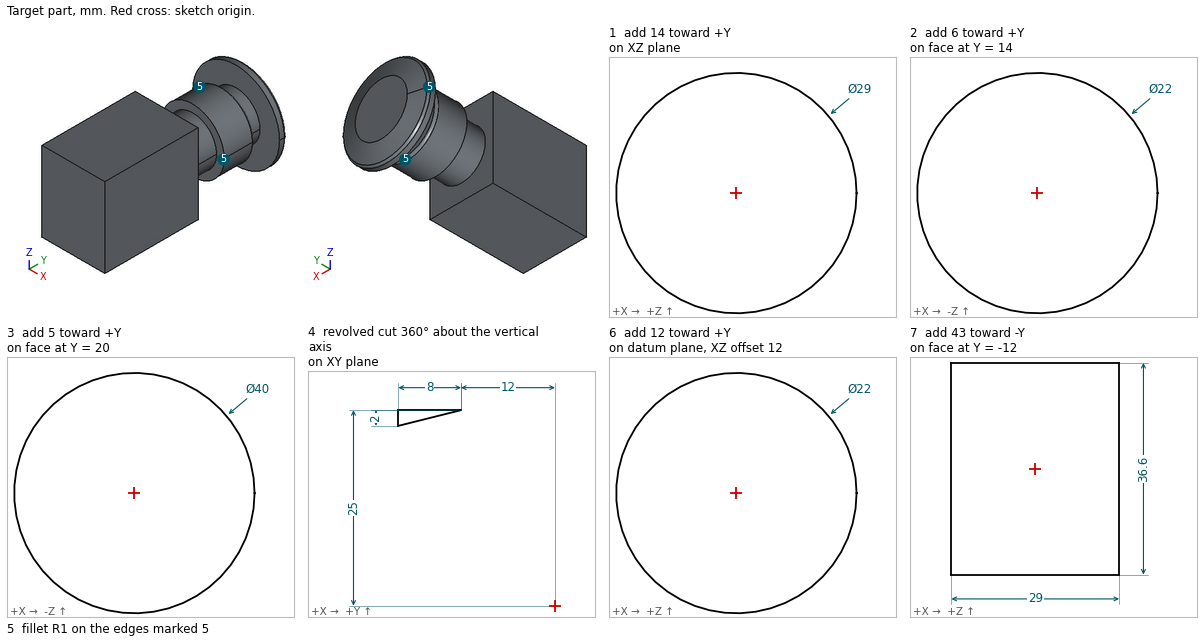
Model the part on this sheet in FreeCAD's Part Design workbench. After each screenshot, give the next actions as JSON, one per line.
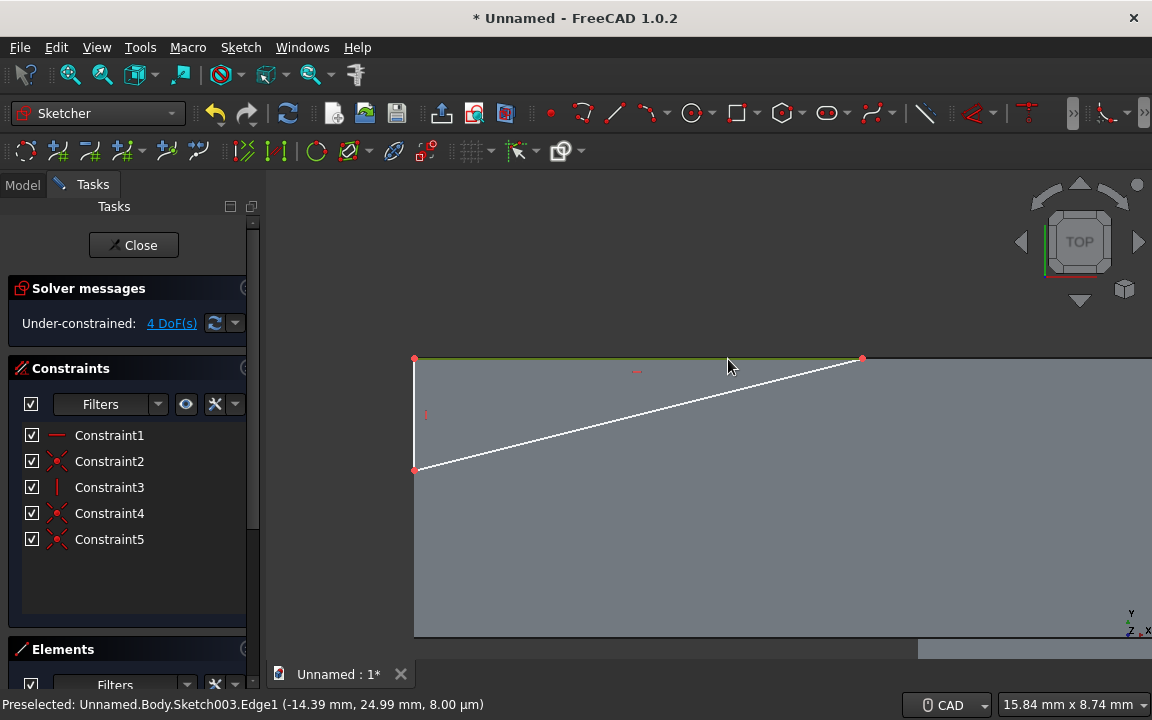
{"action": "key", "text": "l"}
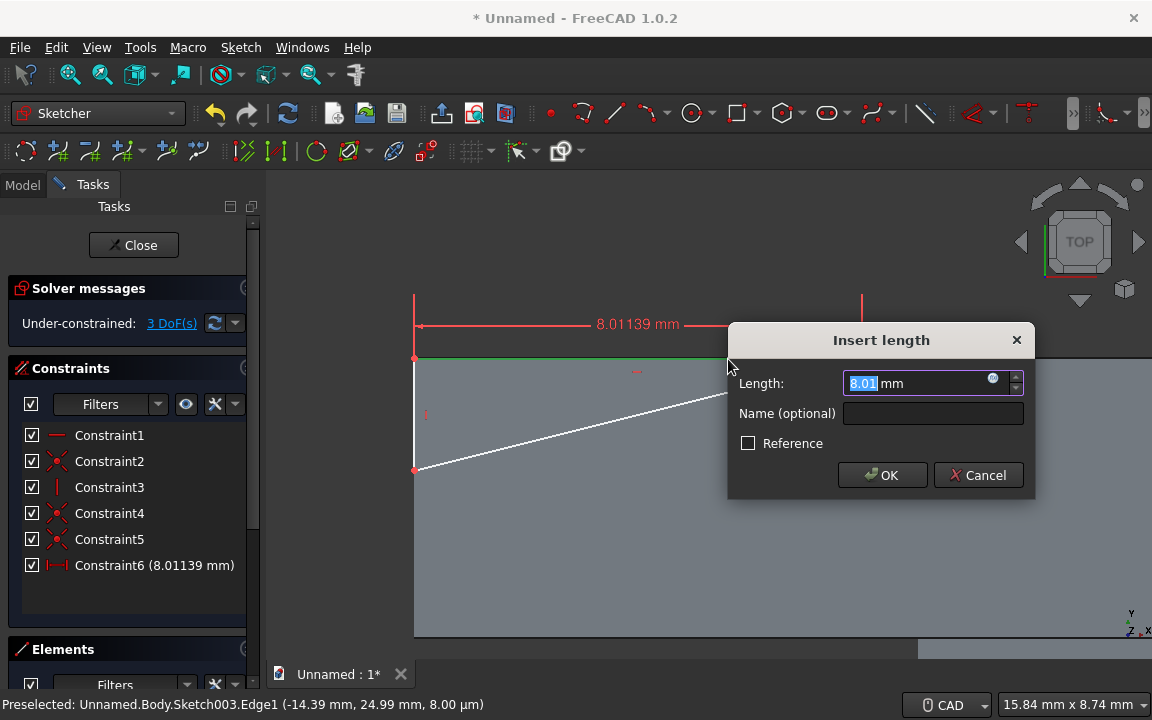
{"action": "type", "text": "8"}
{"action": "key", "text": "Return"}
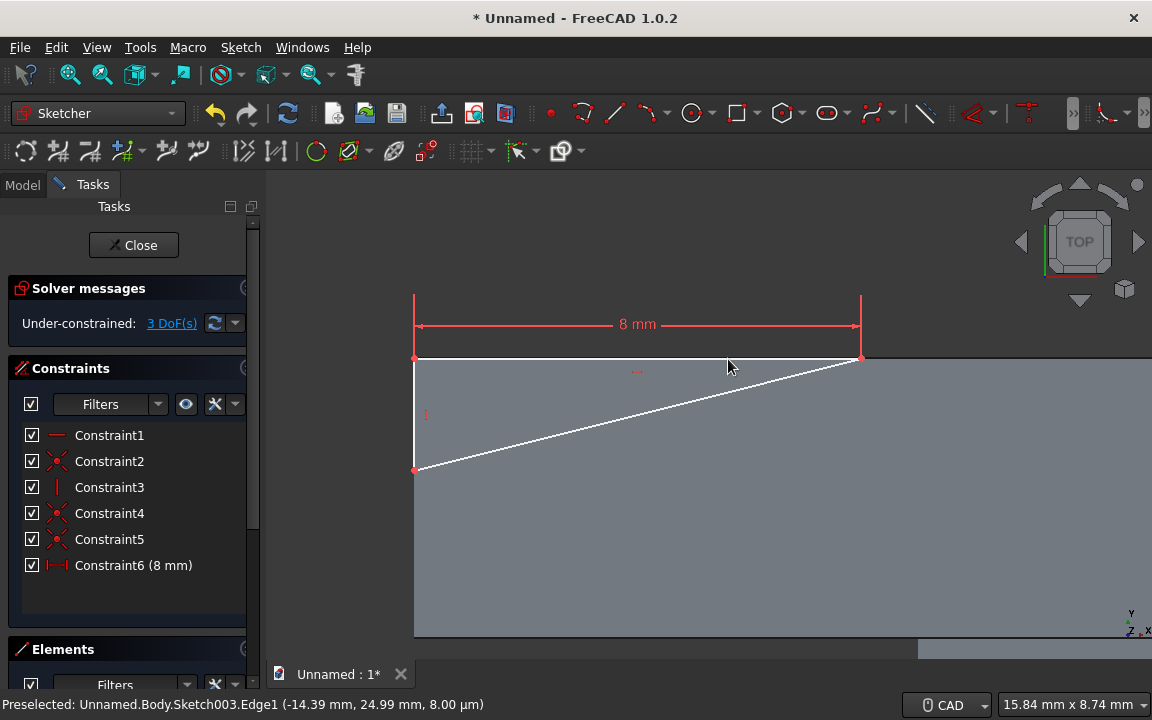
{"action": "left_click", "coordinate": [414, 393]}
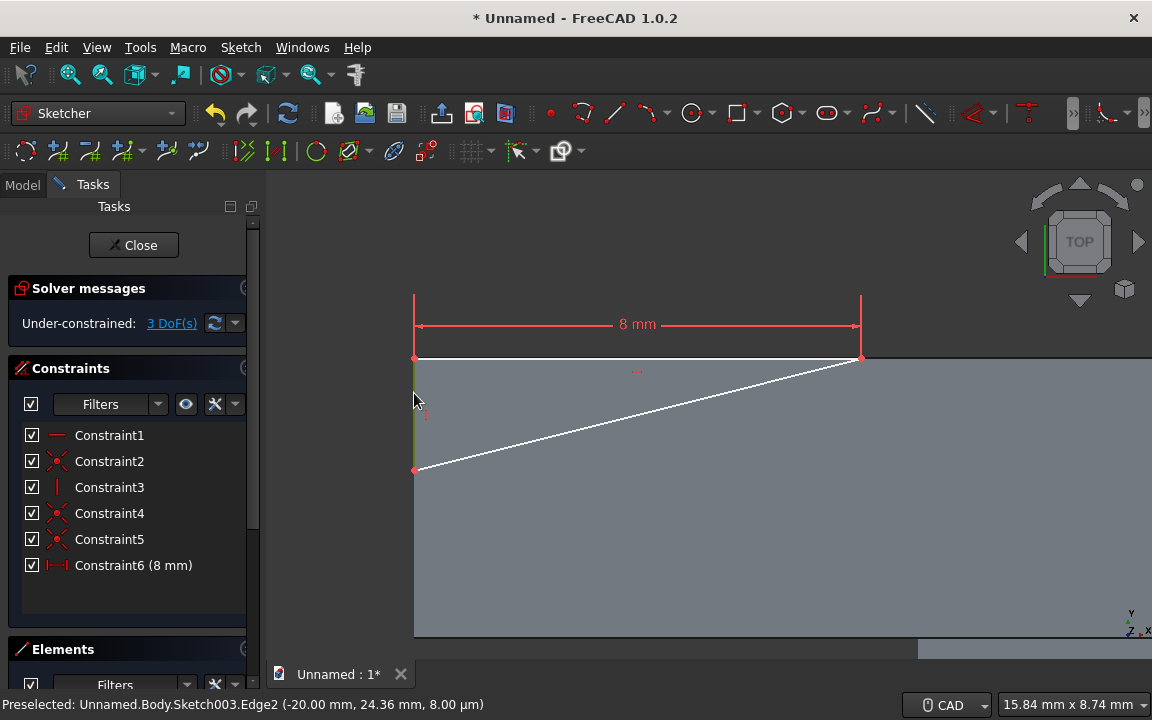
{"action": "key", "text": "i"}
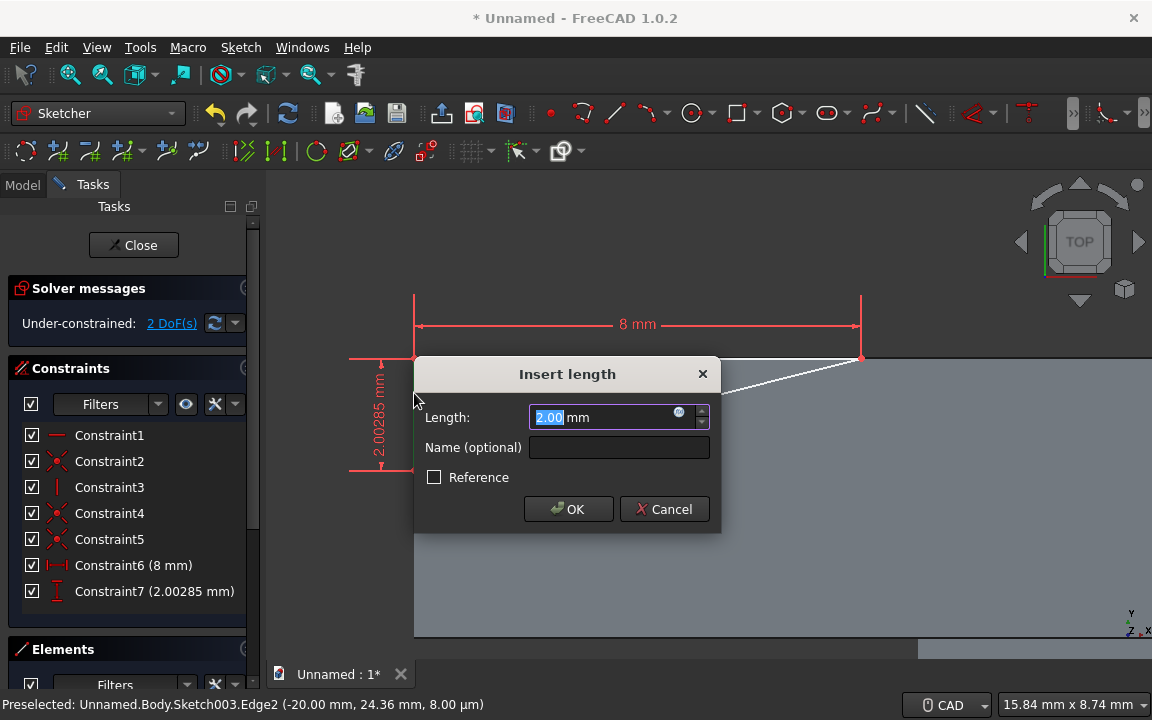
{"action": "type", "text": "2"}
{"action": "key", "text": "Return"}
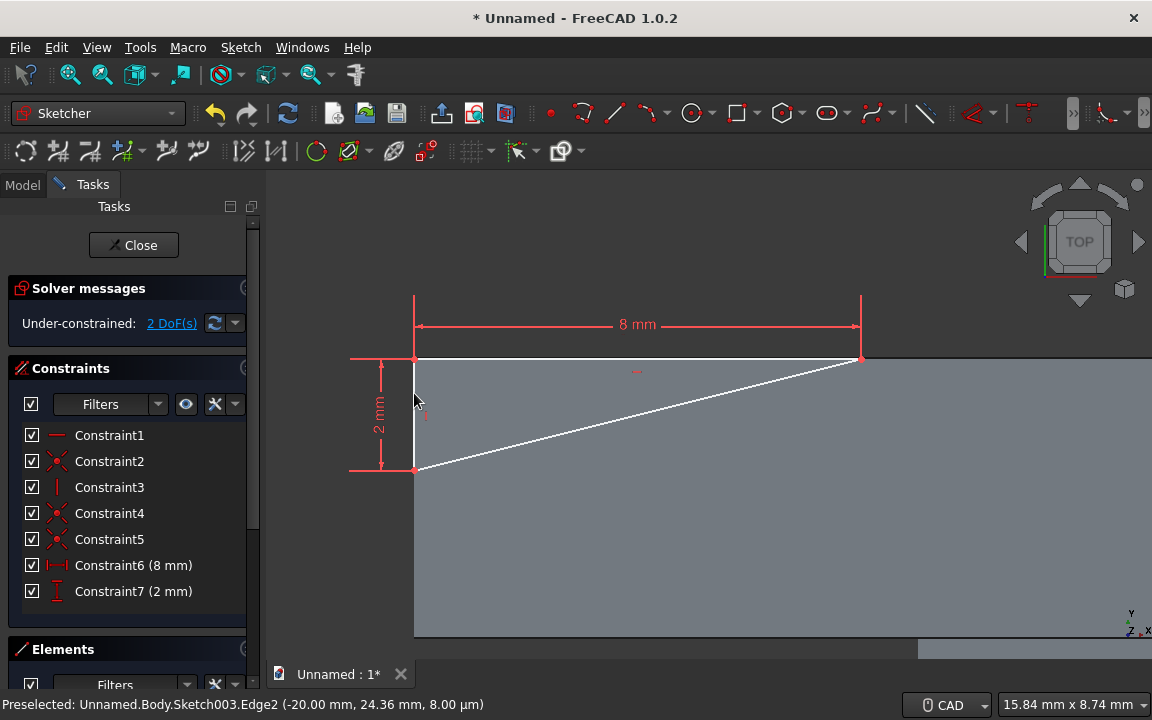
{"action": "left_click", "coordinate": [861, 359]}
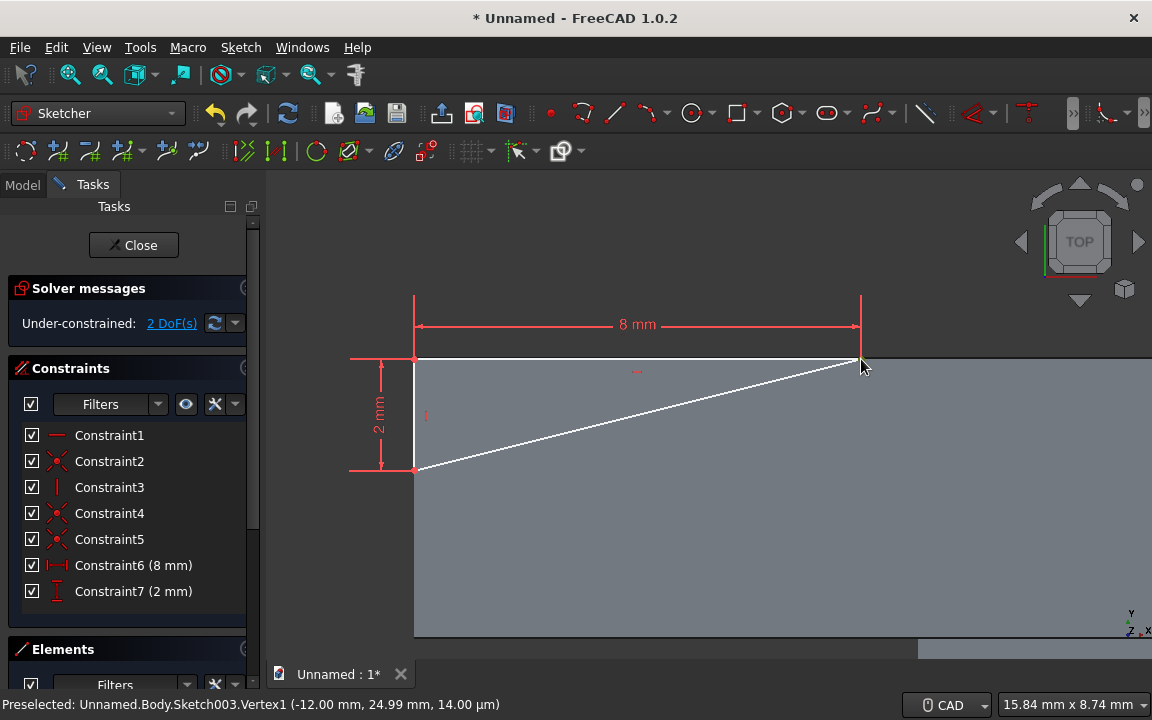
{"action": "key", "text": "l"}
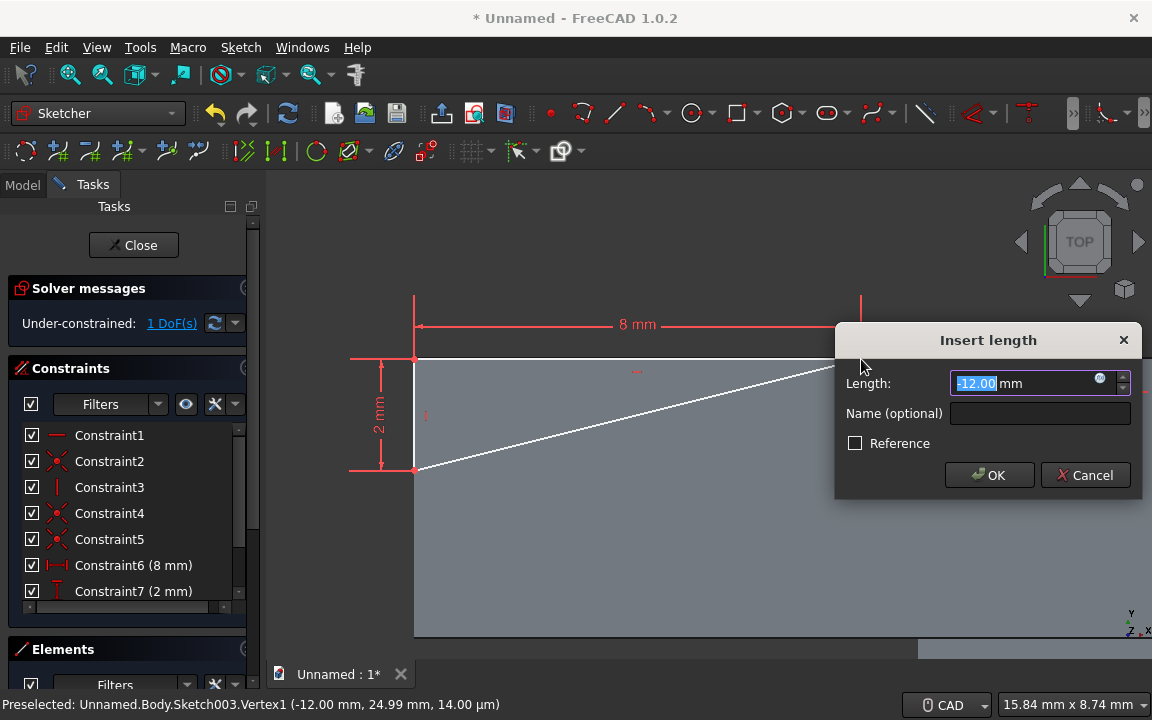
{"action": "type", "text": "-12"}
{"action": "key", "text": "Return"}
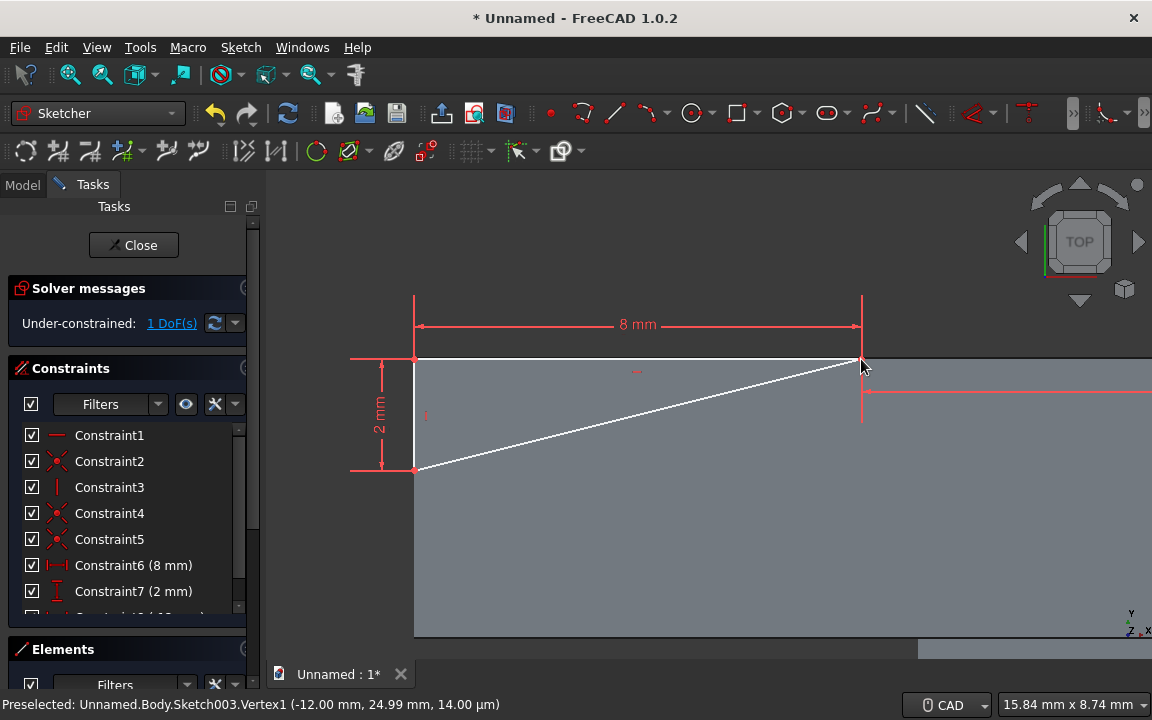
{"action": "left_click", "coordinate": [862, 359]}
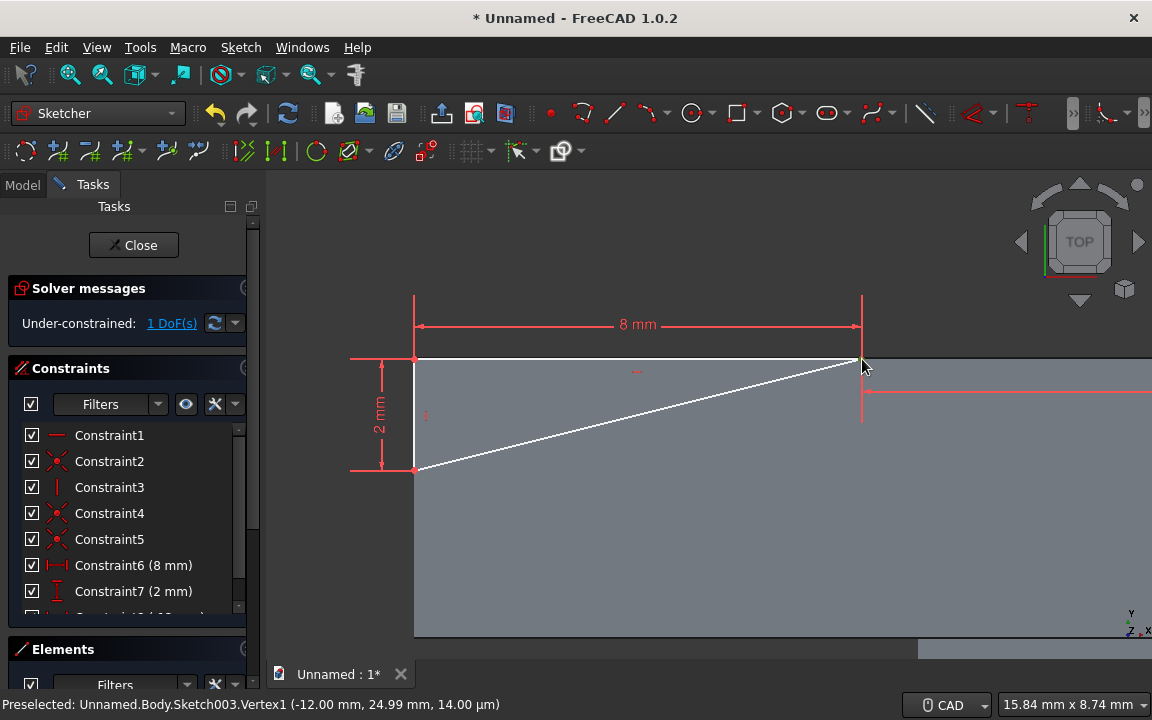
{"action": "left_click", "coordinate": [996, 114]}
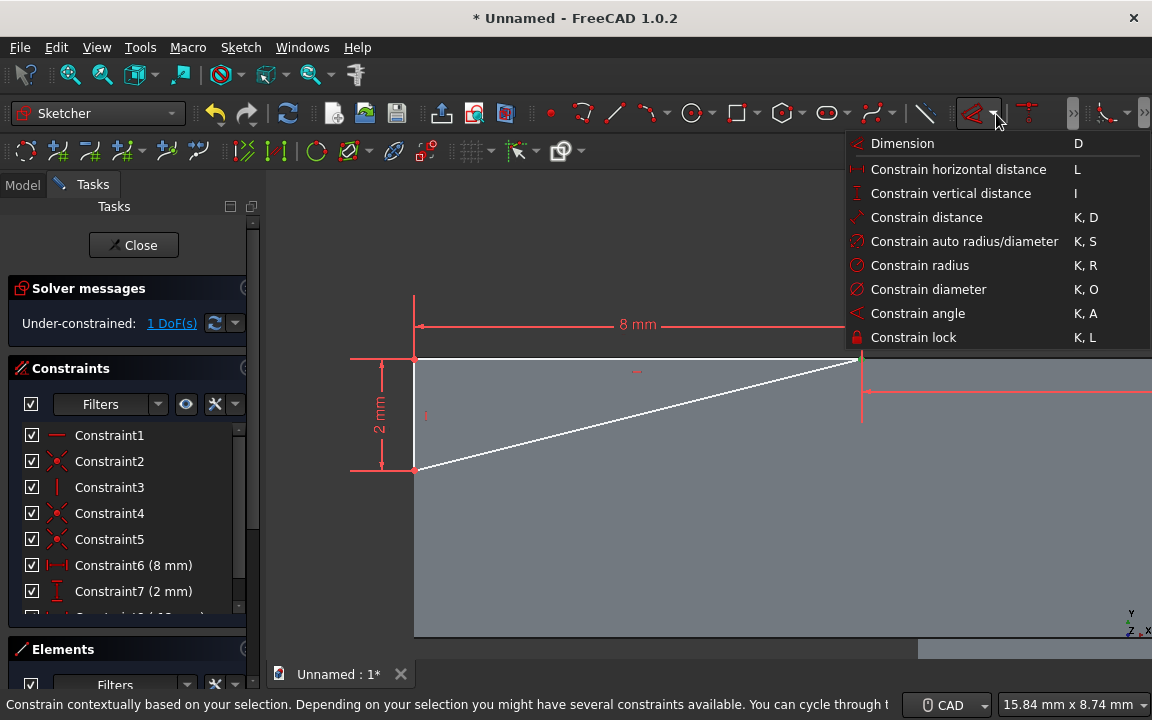
{"action": "left_click", "coordinate": [998, 193]}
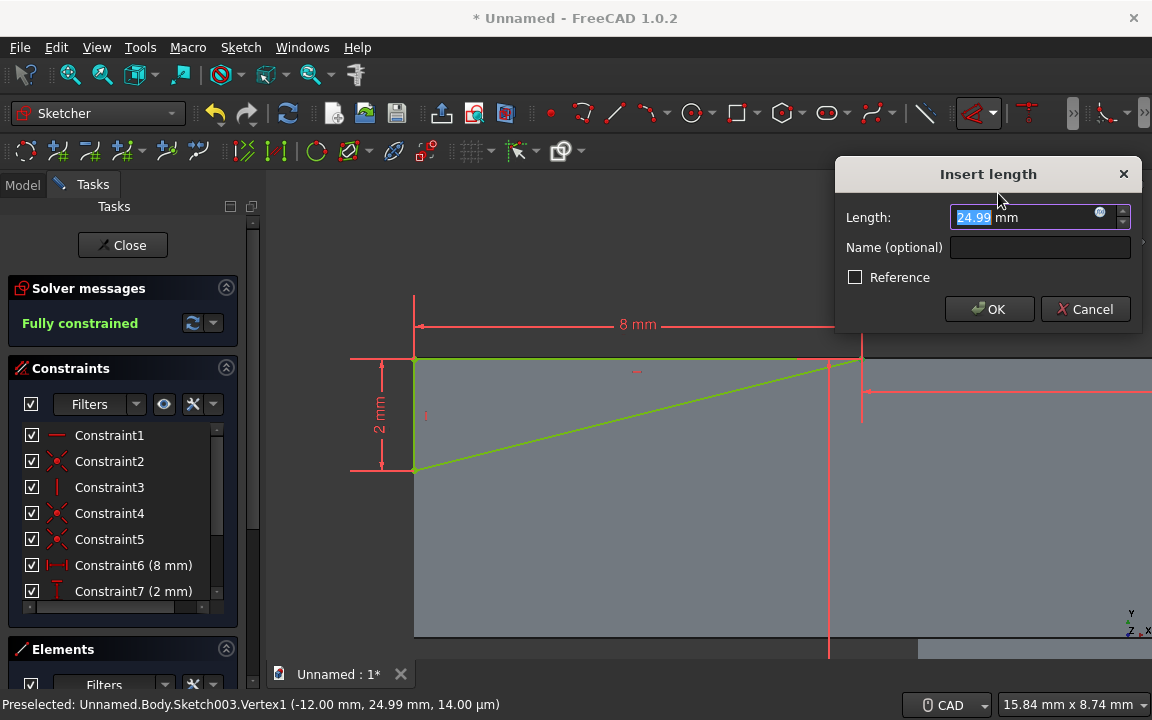
{"action": "type", "text": "25"}
{"action": "key", "text": "Return"}